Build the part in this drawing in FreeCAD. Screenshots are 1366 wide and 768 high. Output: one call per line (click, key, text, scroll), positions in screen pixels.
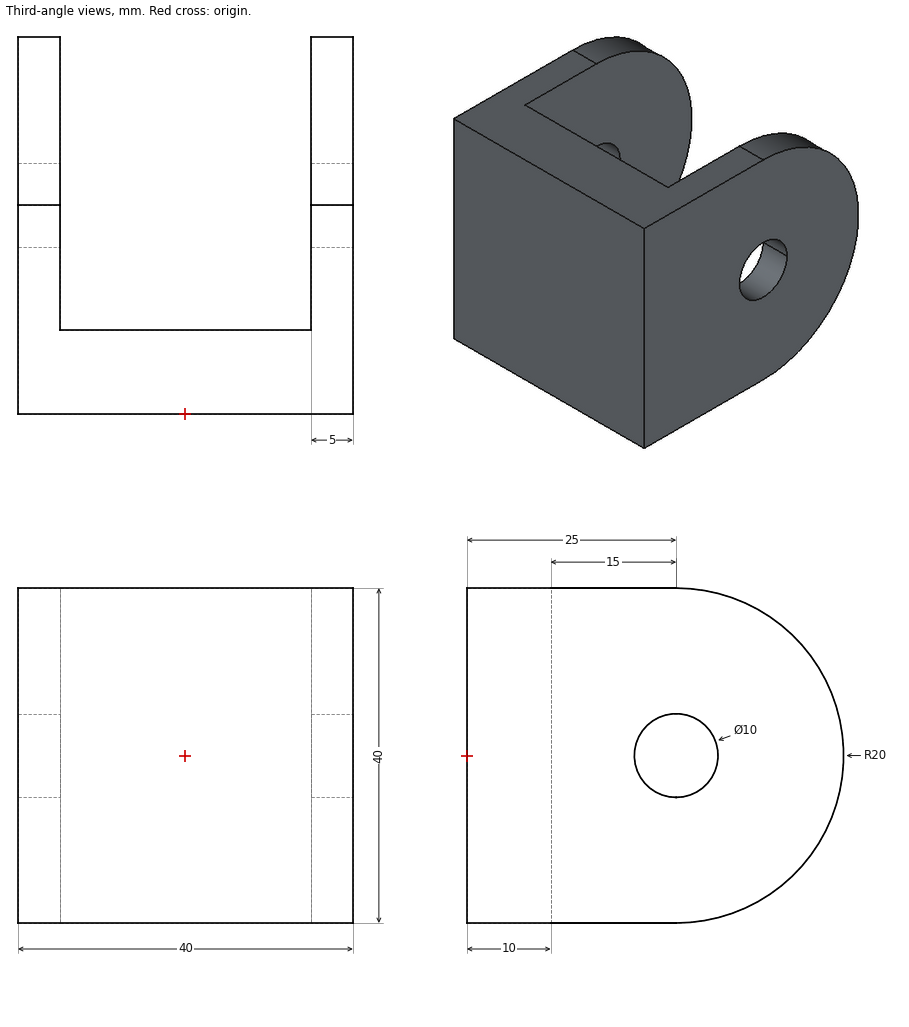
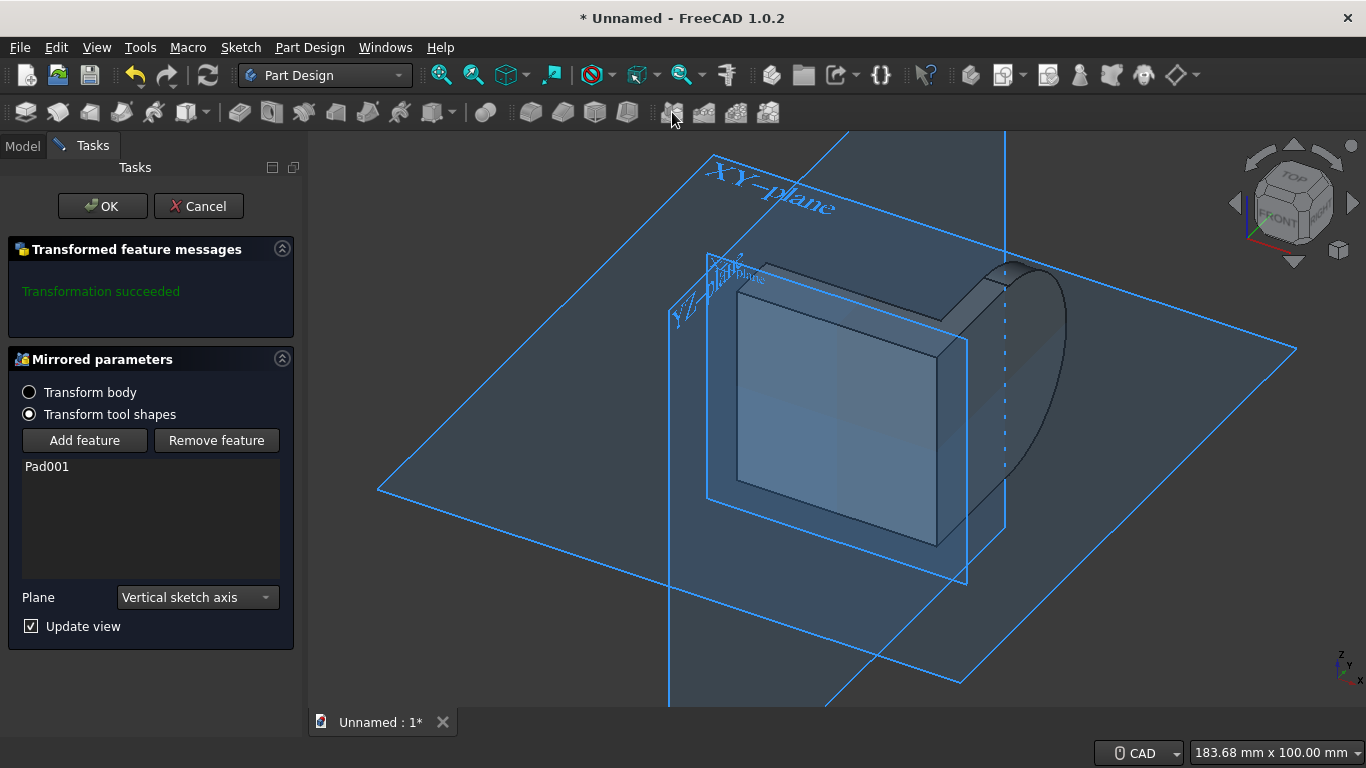
click(198, 598)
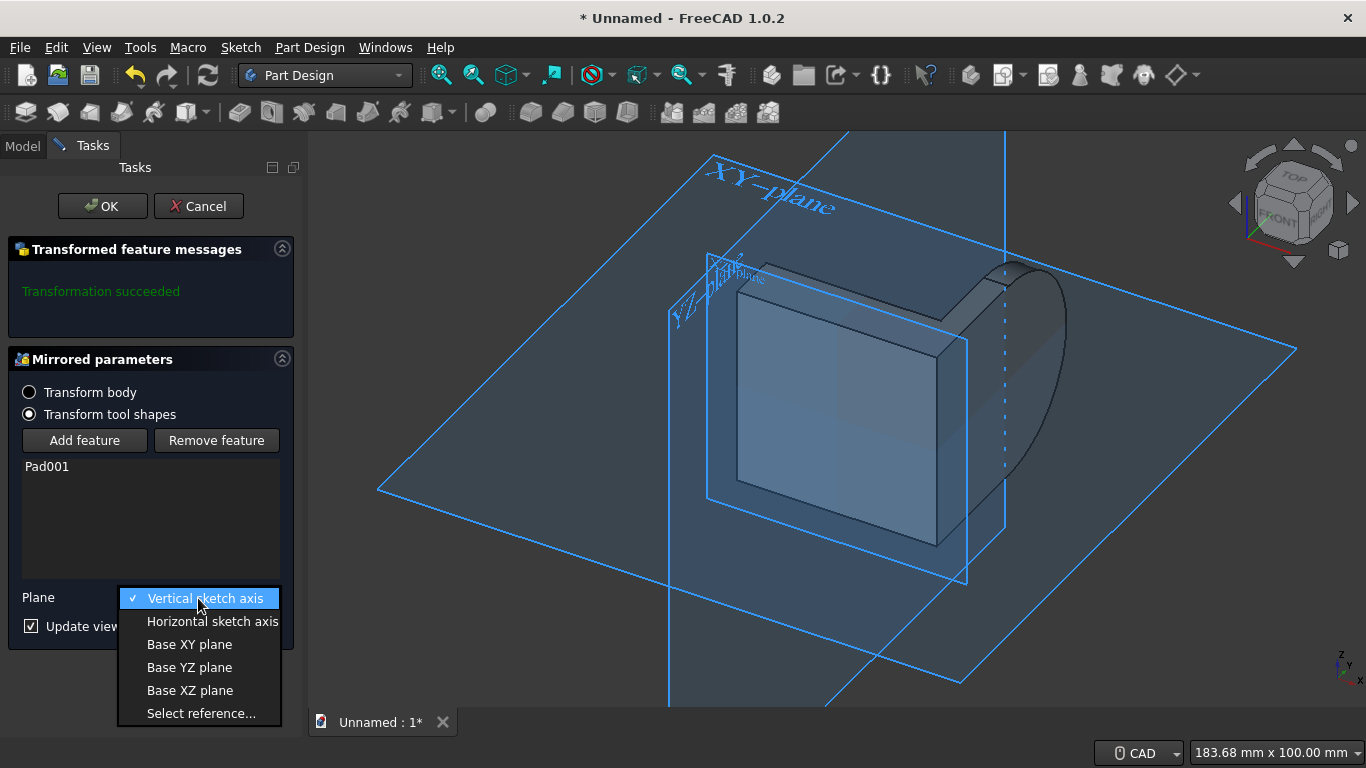
click(198, 668)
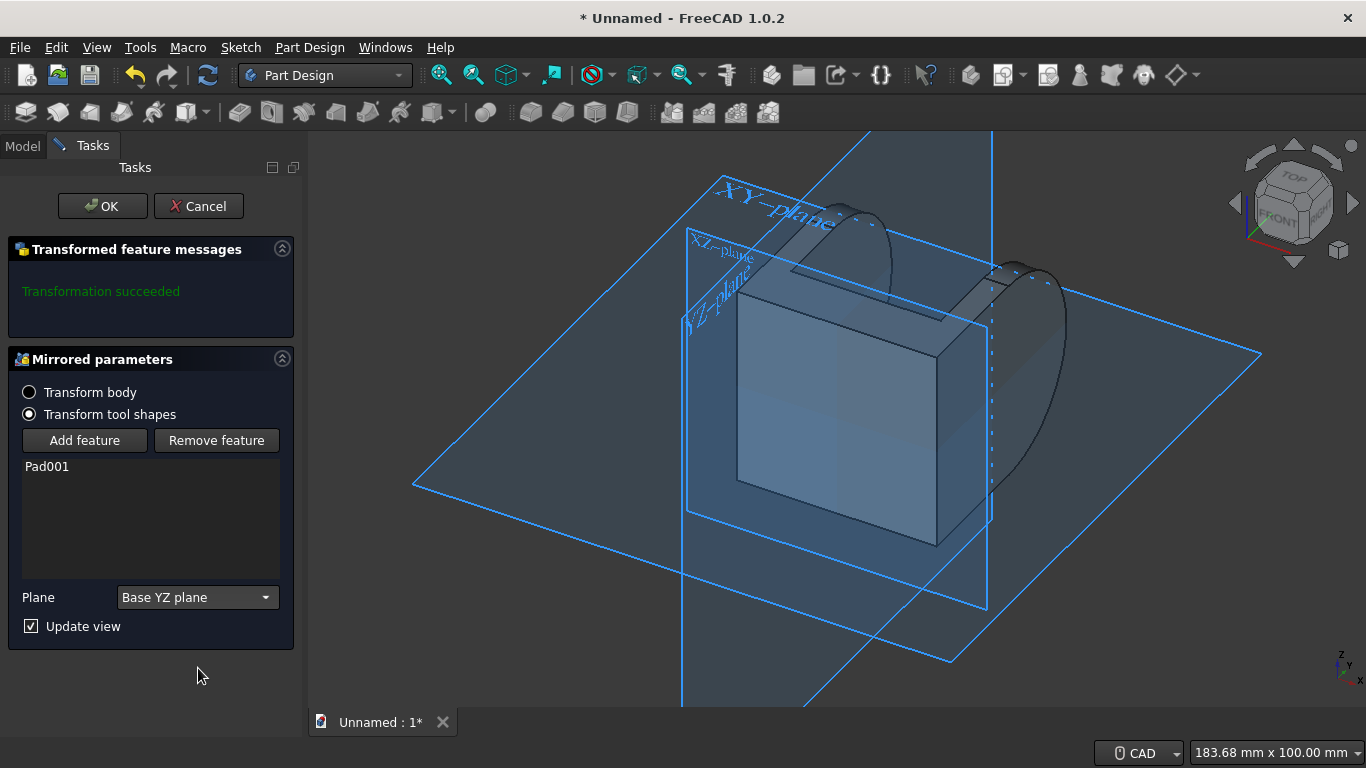
click(103, 206)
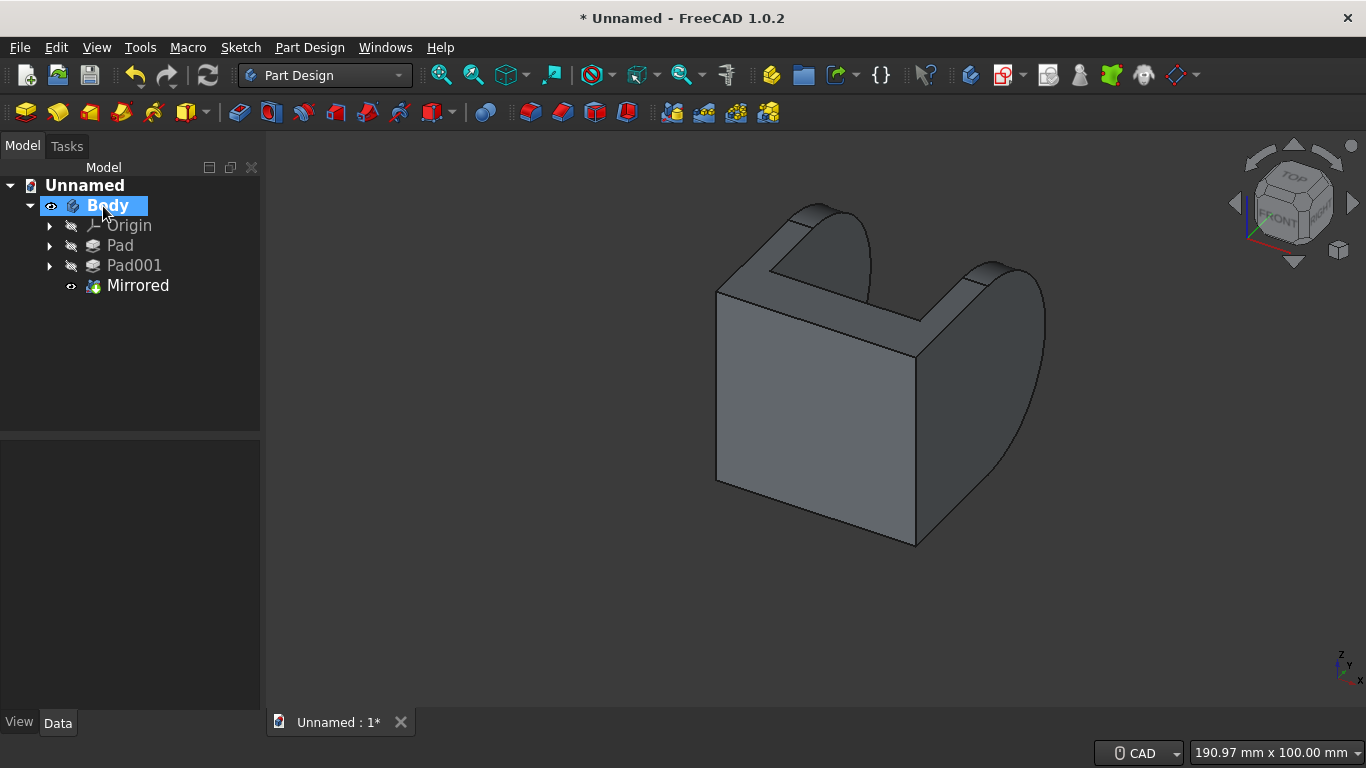
click(50, 226)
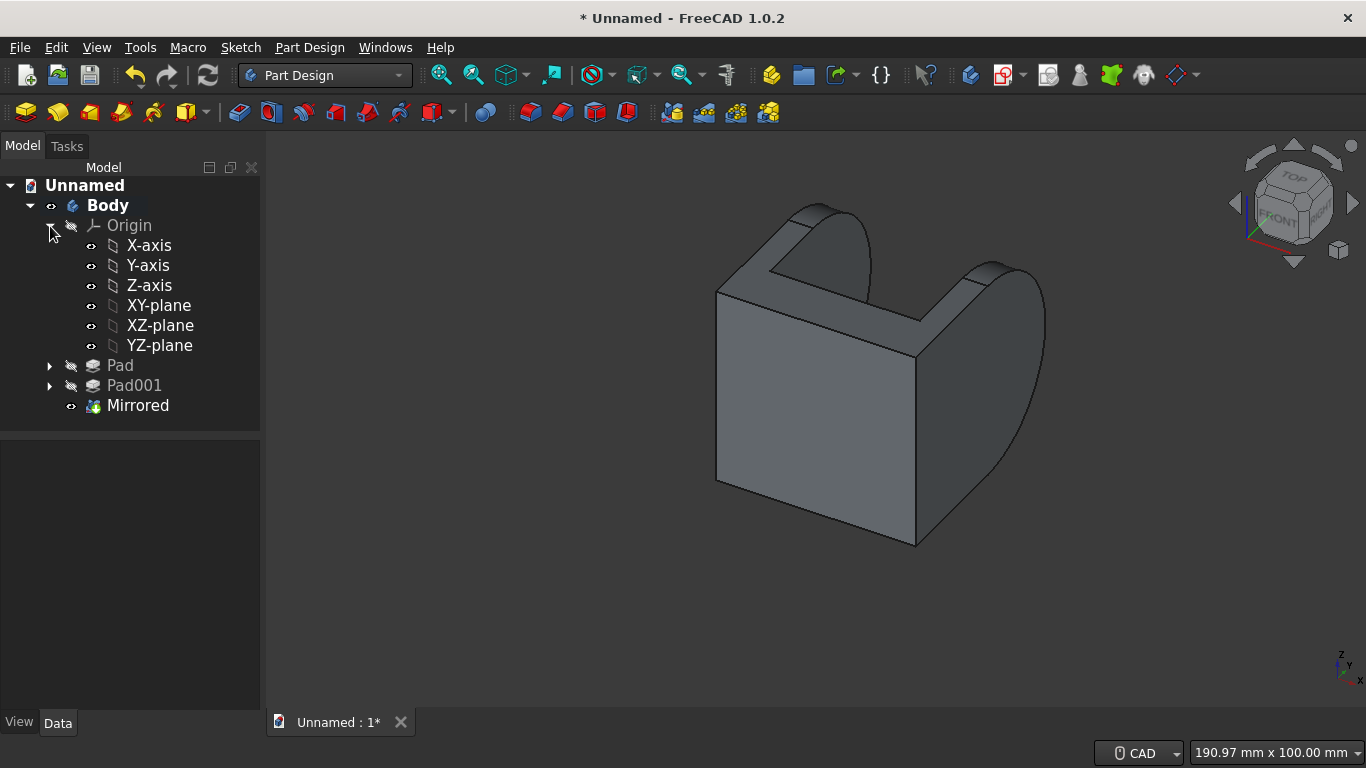
click(136, 346)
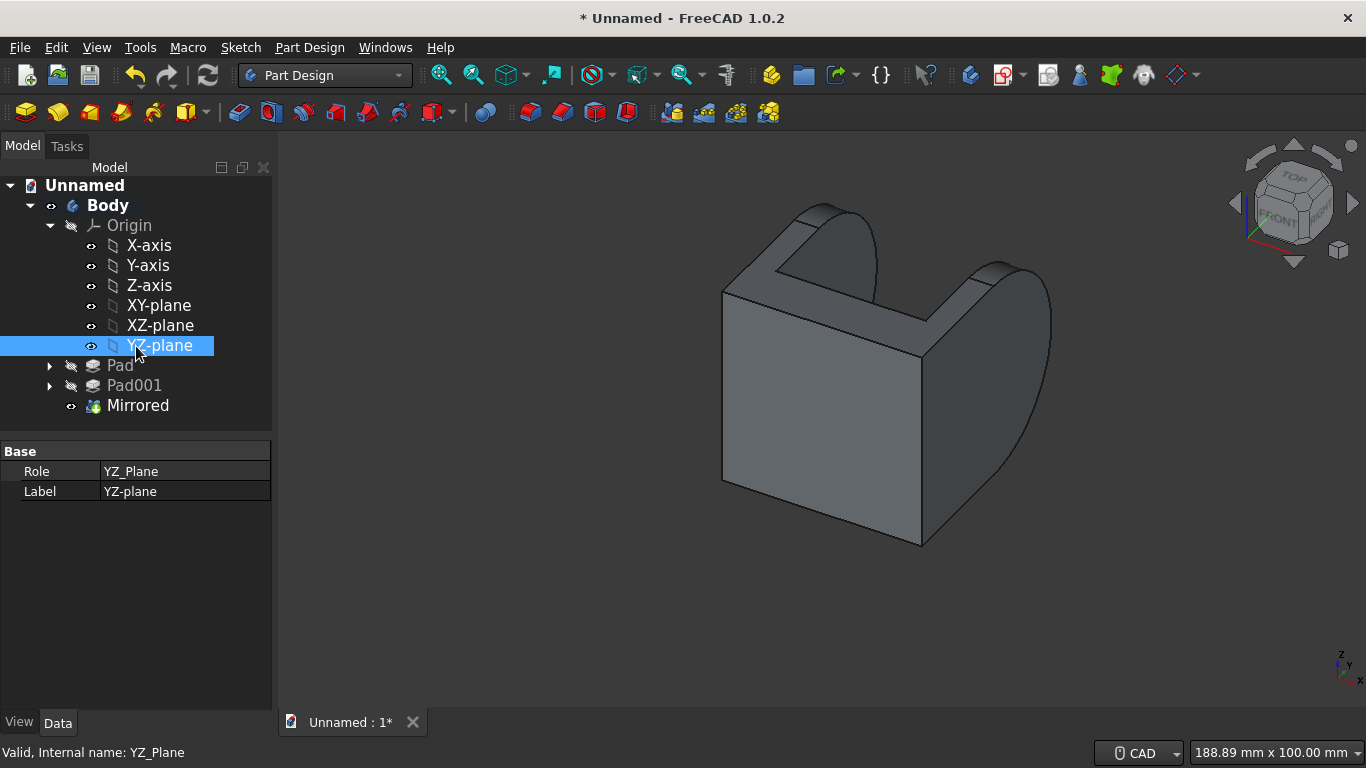
click(1176, 76)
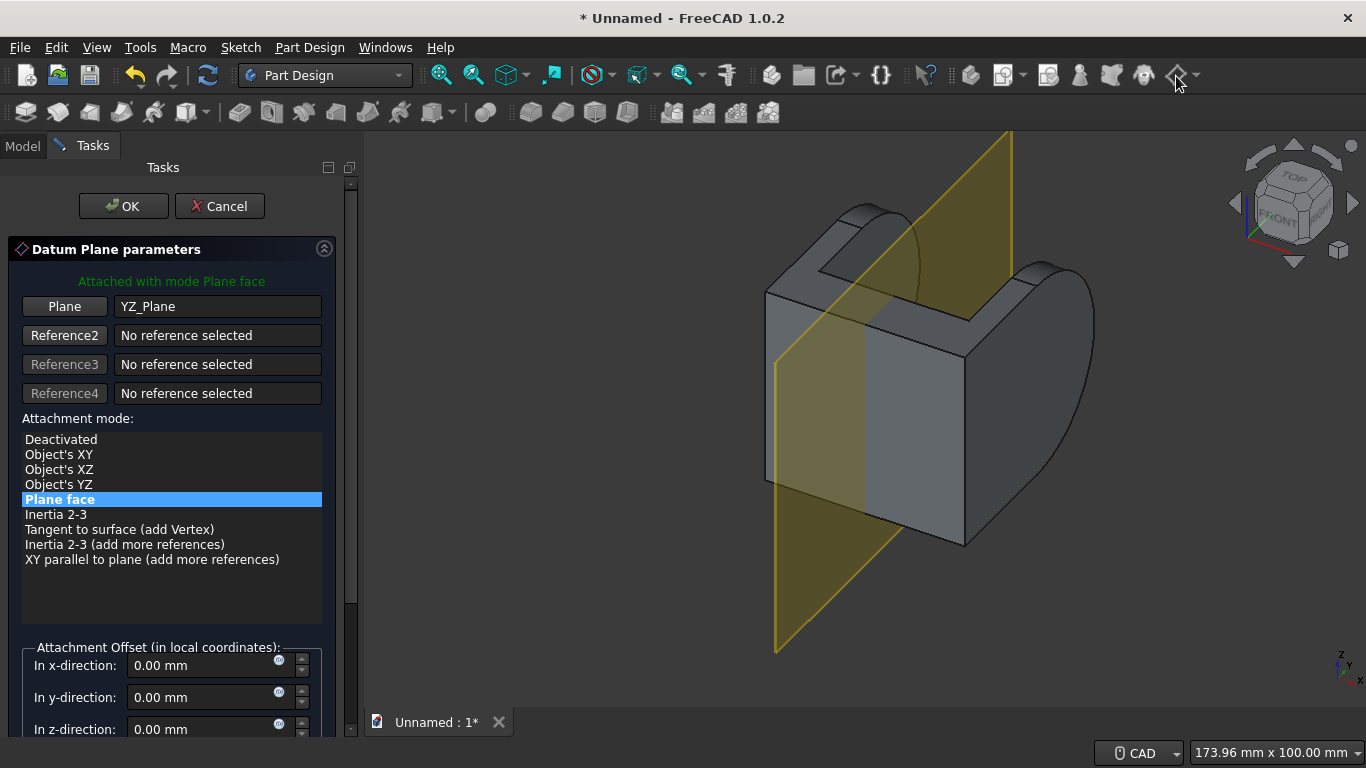
scroll(351, 456, down, 2)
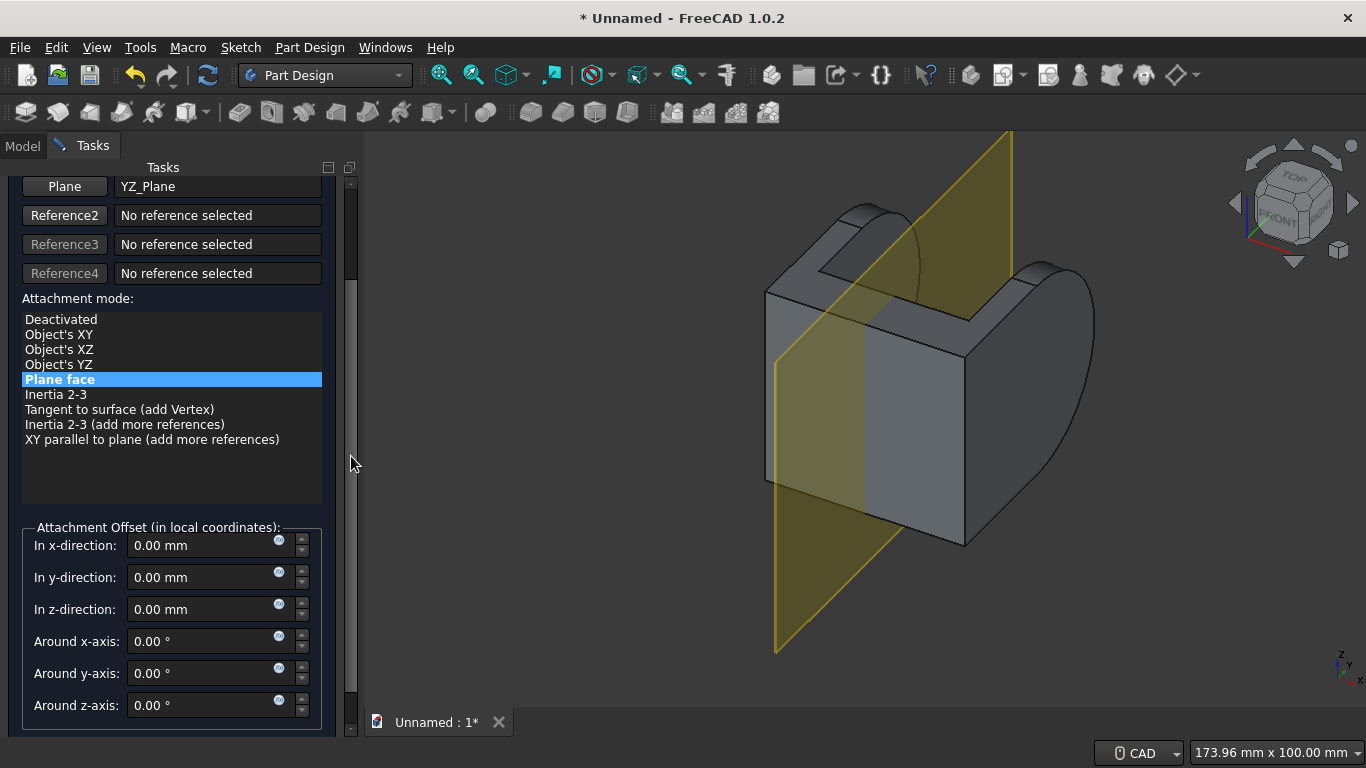
triple_click(210, 609)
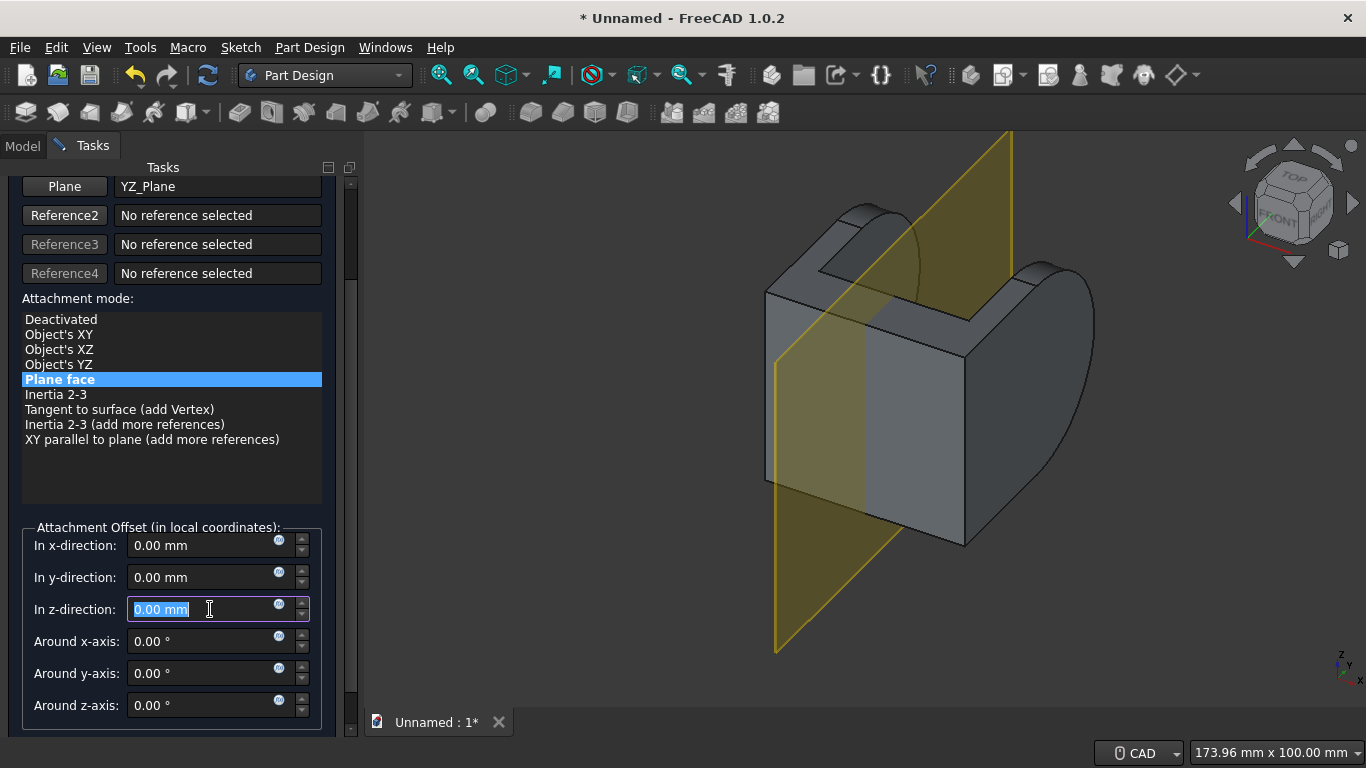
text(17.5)
key(Tab)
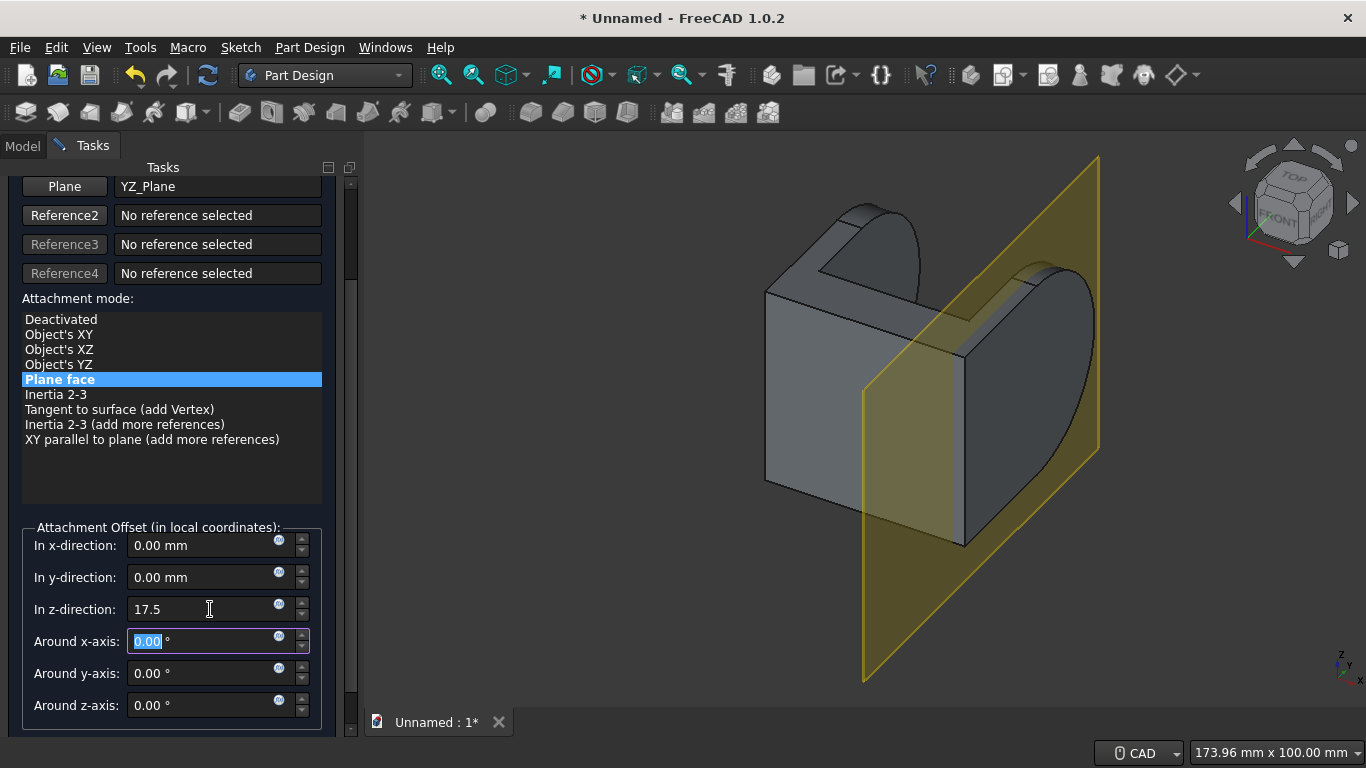
scroll(351, 456, up, 3)